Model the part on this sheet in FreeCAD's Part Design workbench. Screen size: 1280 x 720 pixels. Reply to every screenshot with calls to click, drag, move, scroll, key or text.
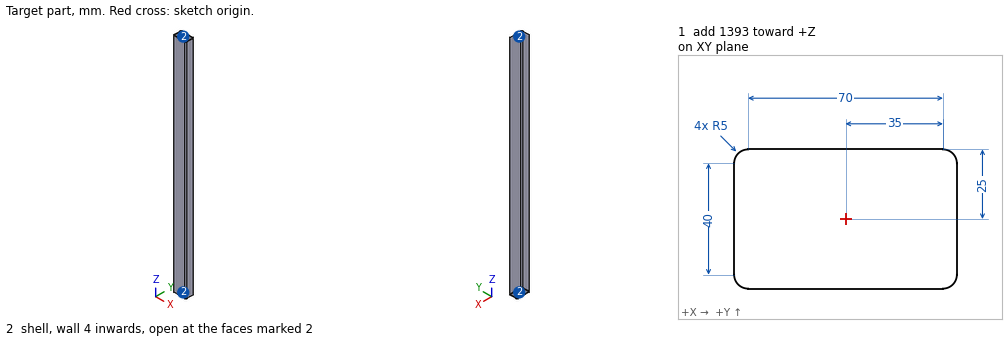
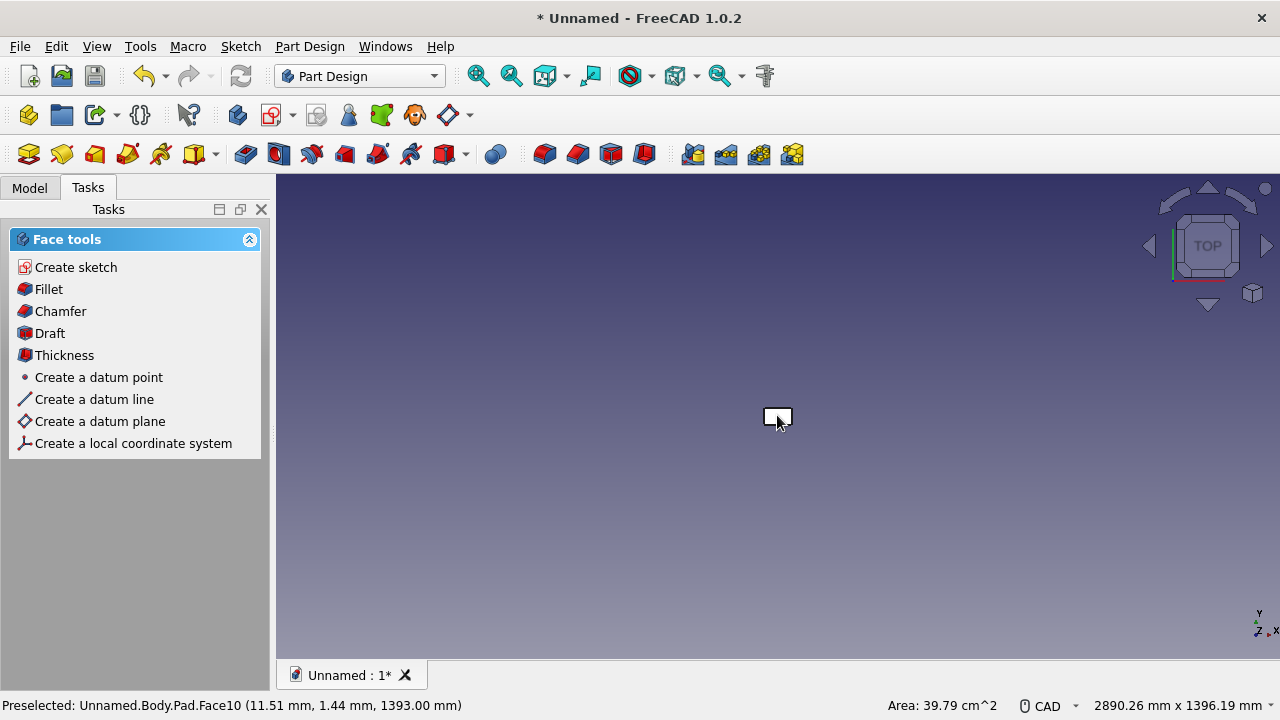
key(1)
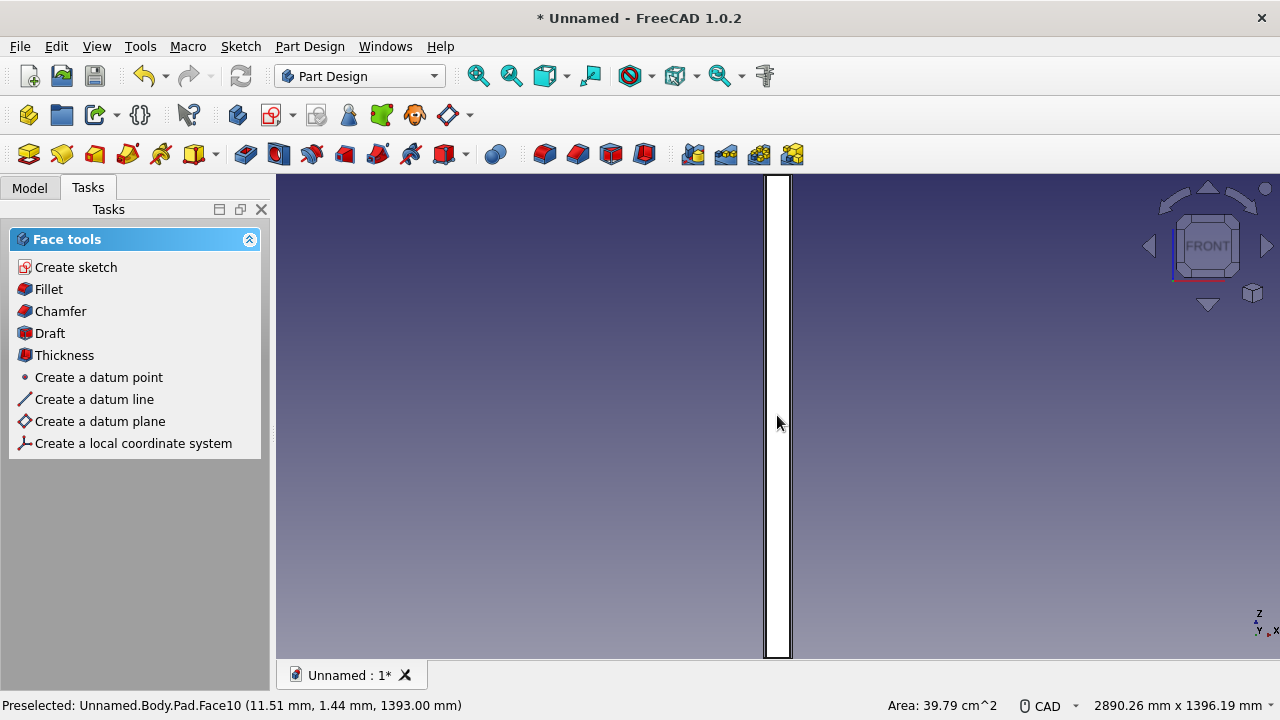
key(3)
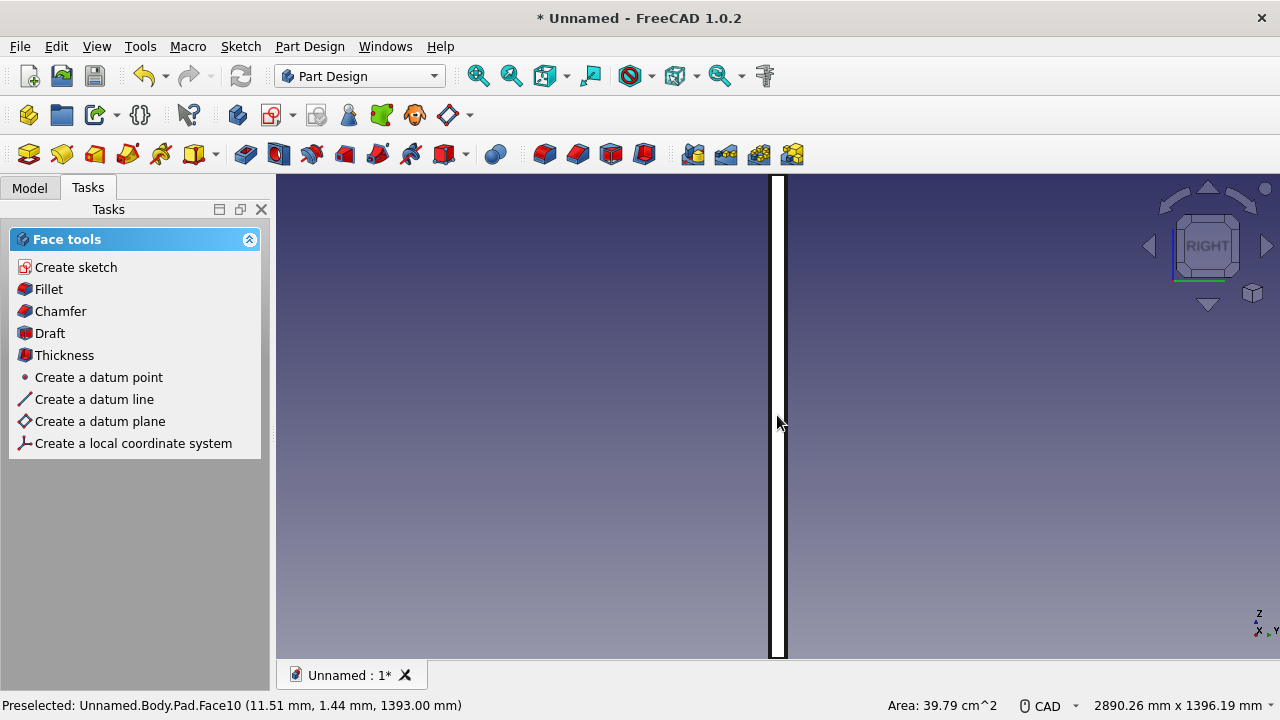
key(5)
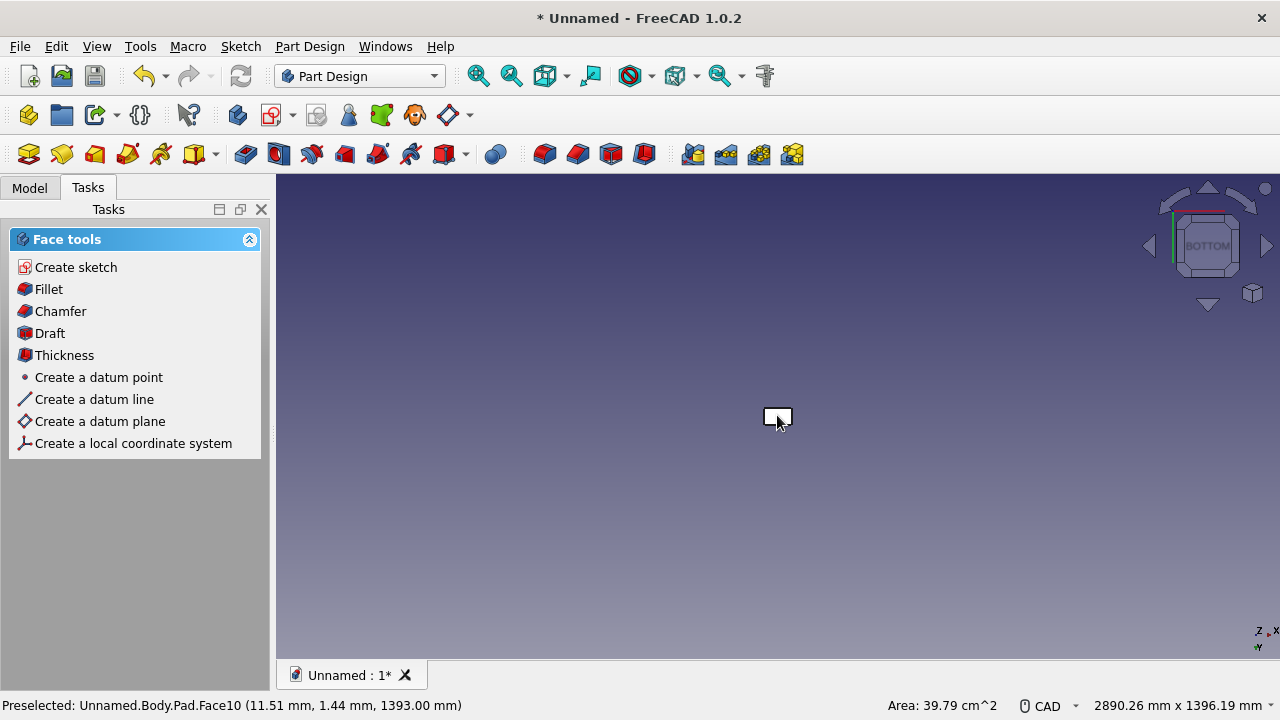
click(479, 76)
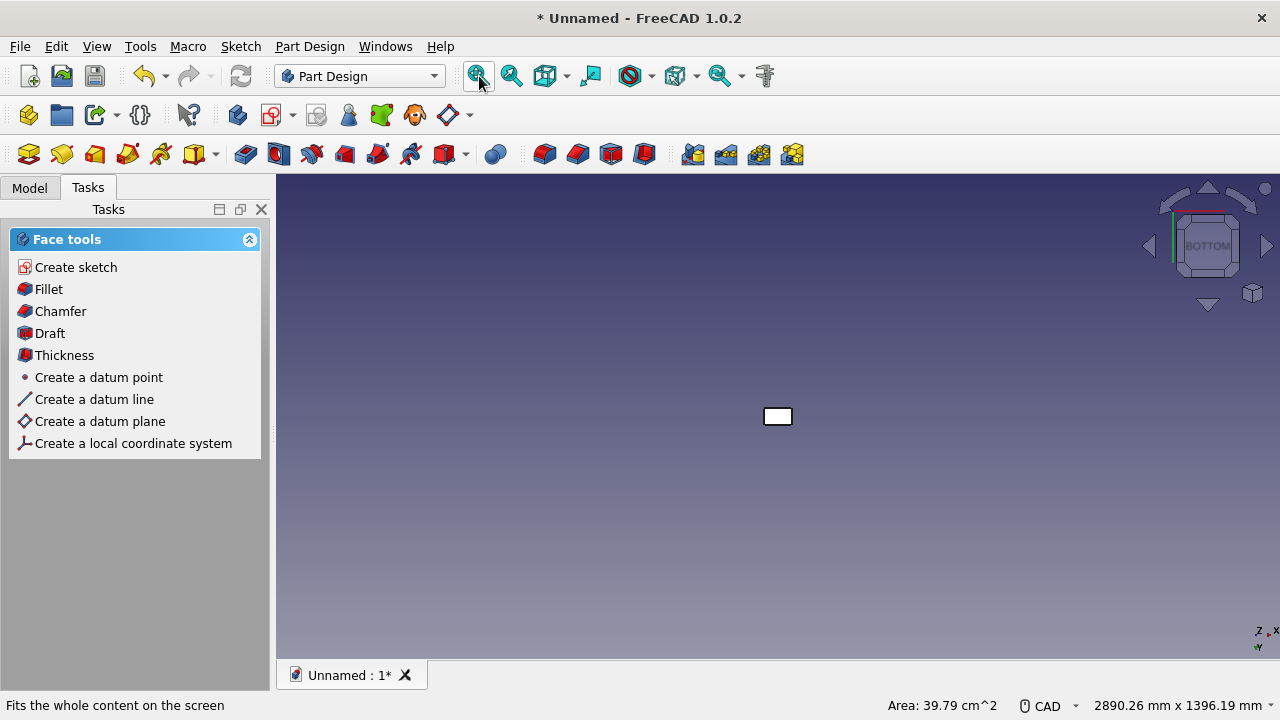
click(782, 415, ctrl)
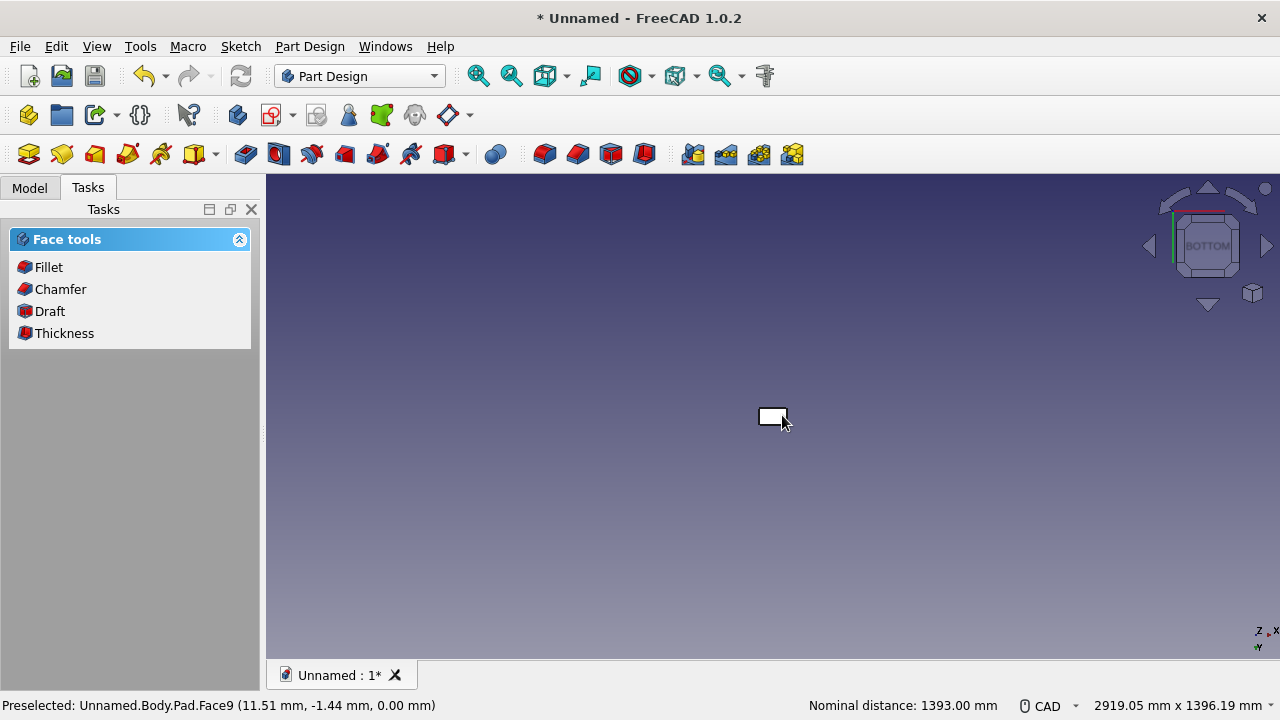
click(644, 154)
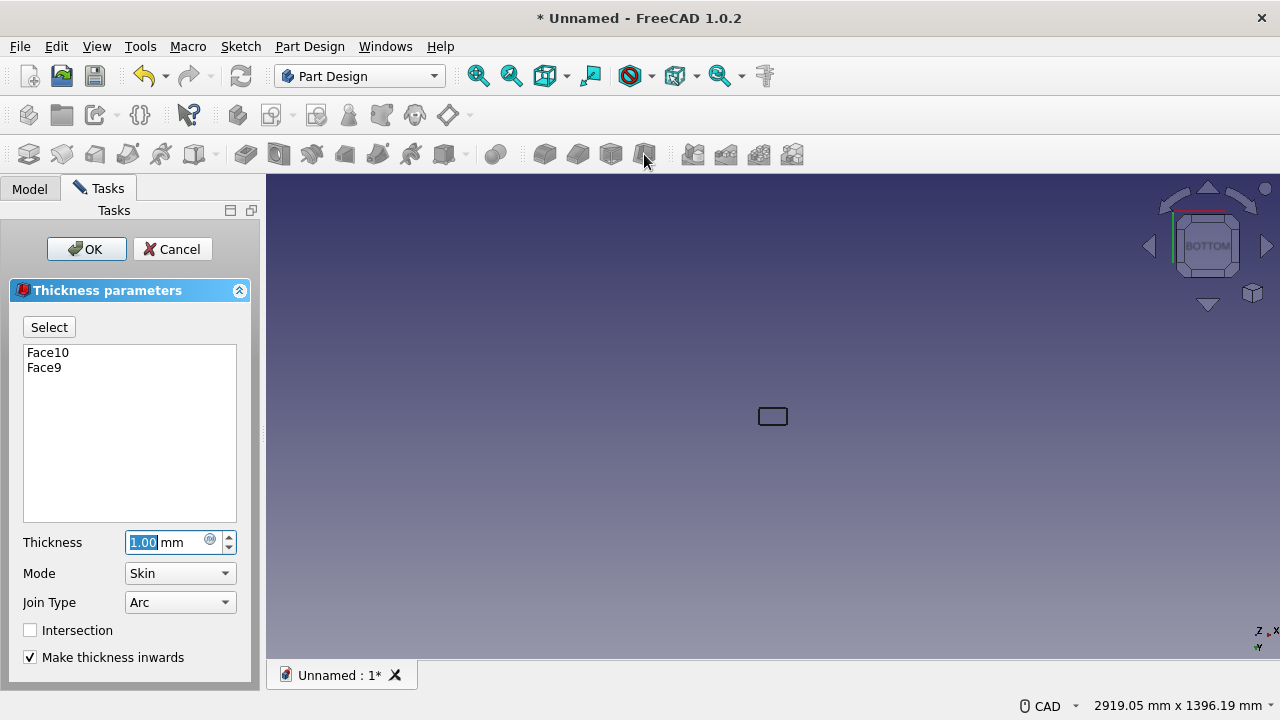
text(4)
key(Tab)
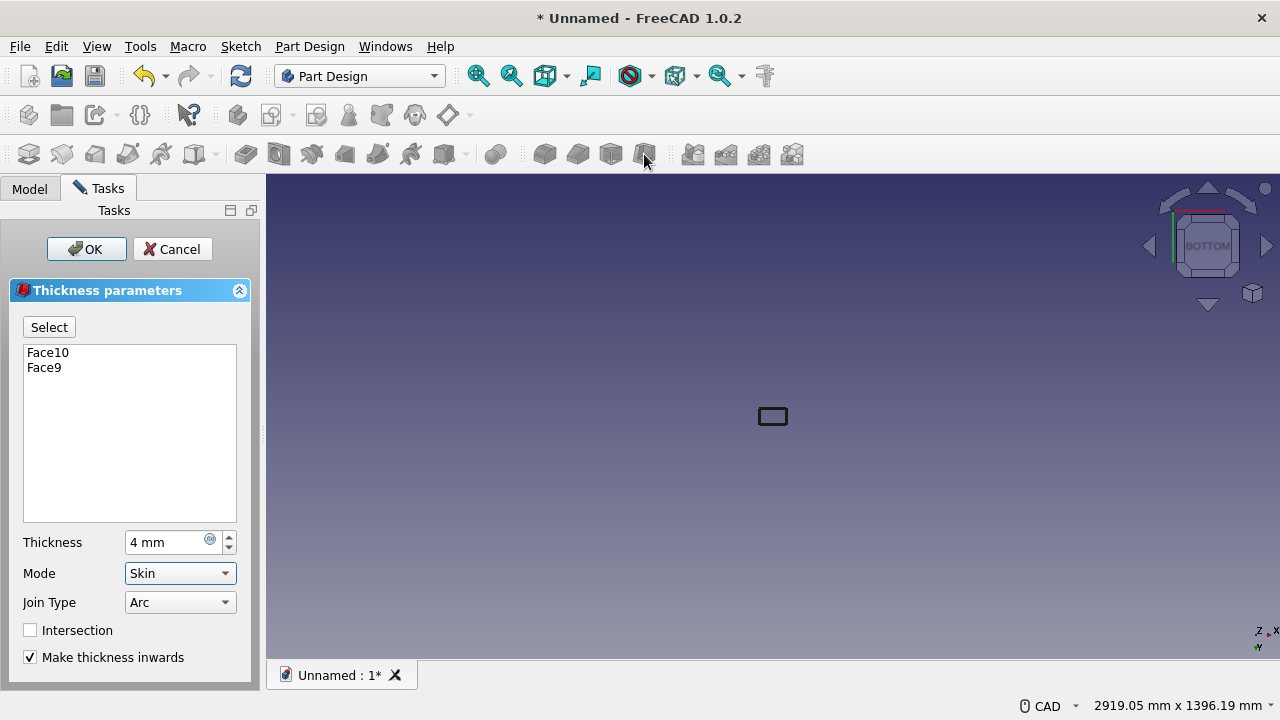
click(181, 602)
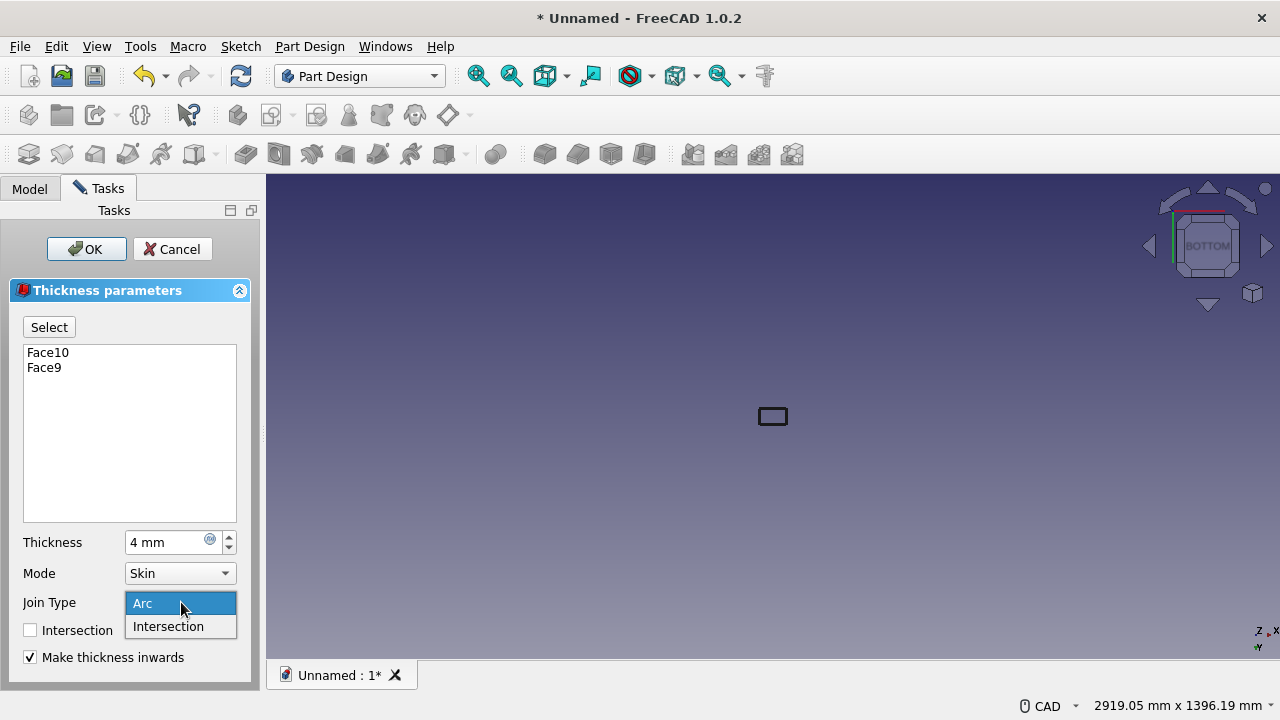
click(179, 626)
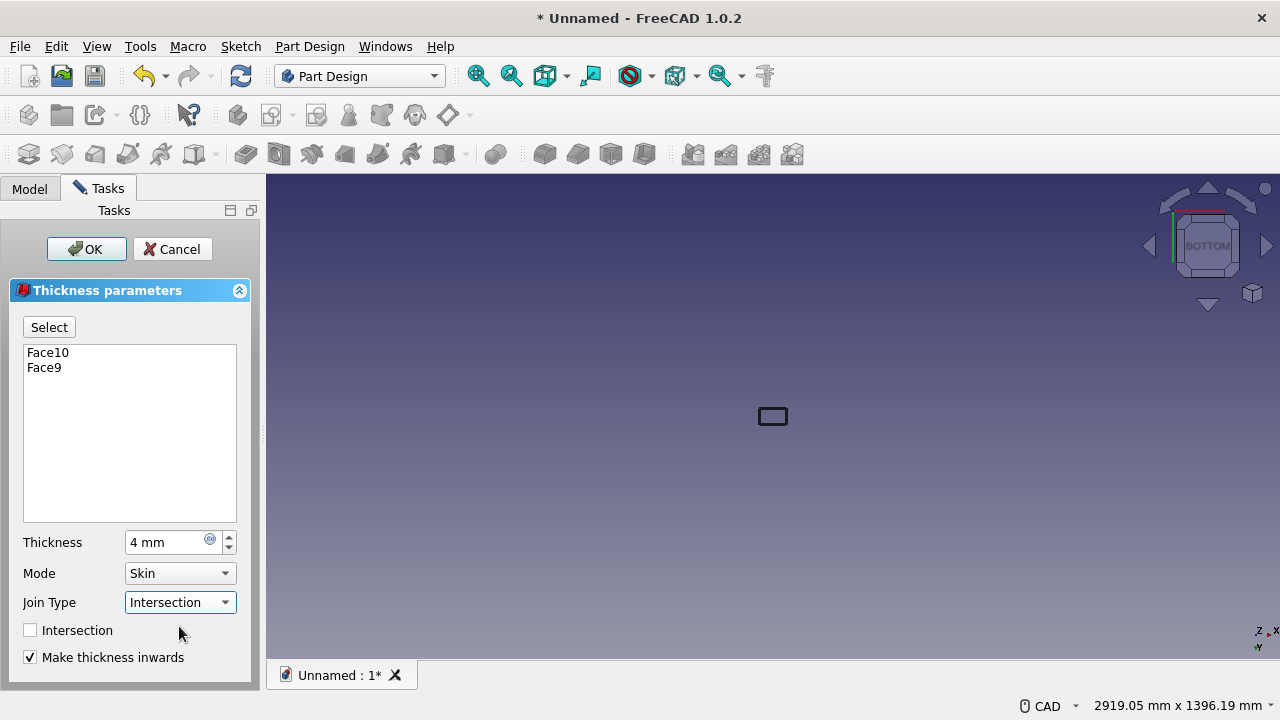
click(87, 249)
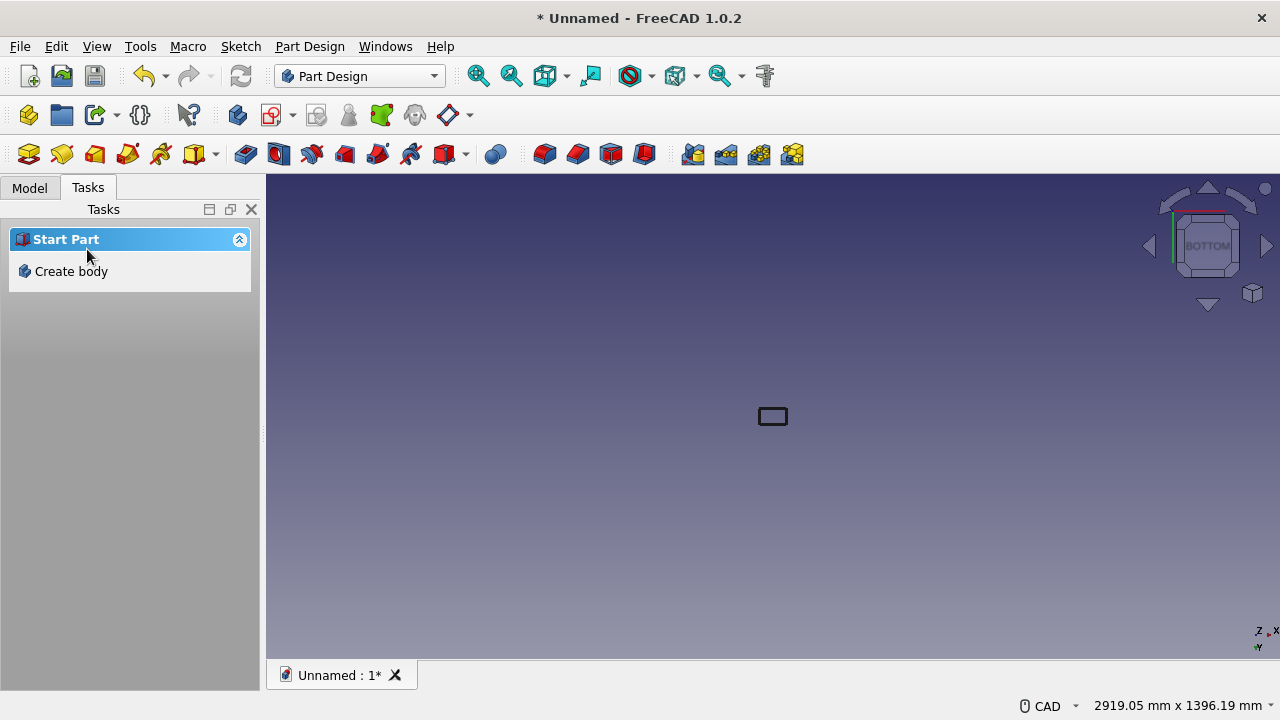
key(0)